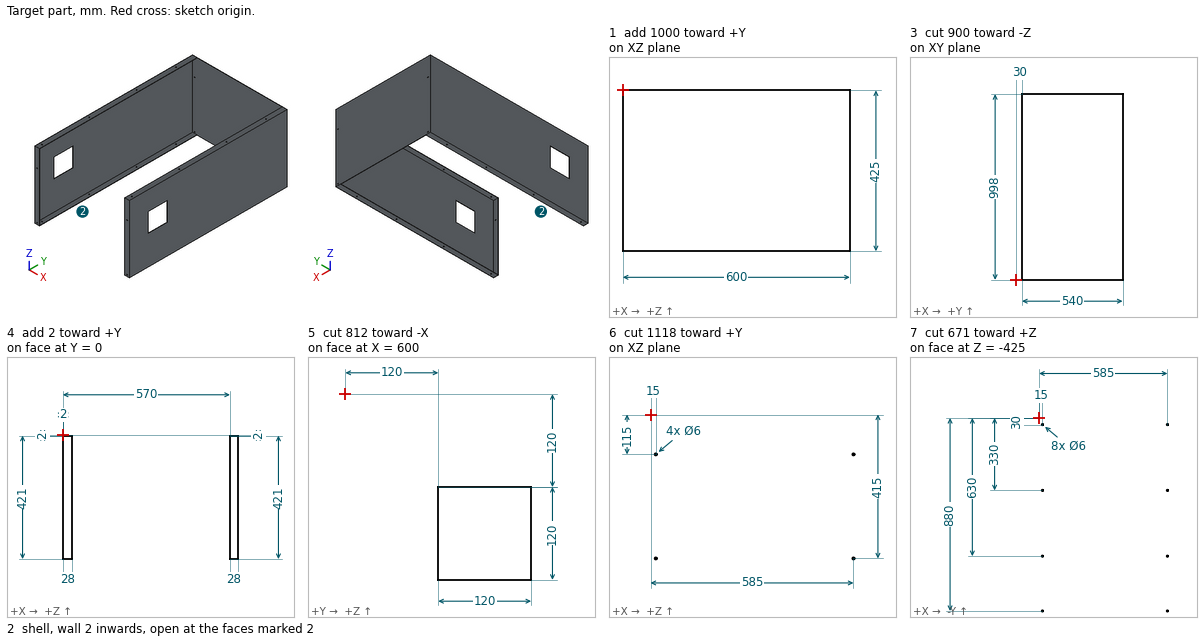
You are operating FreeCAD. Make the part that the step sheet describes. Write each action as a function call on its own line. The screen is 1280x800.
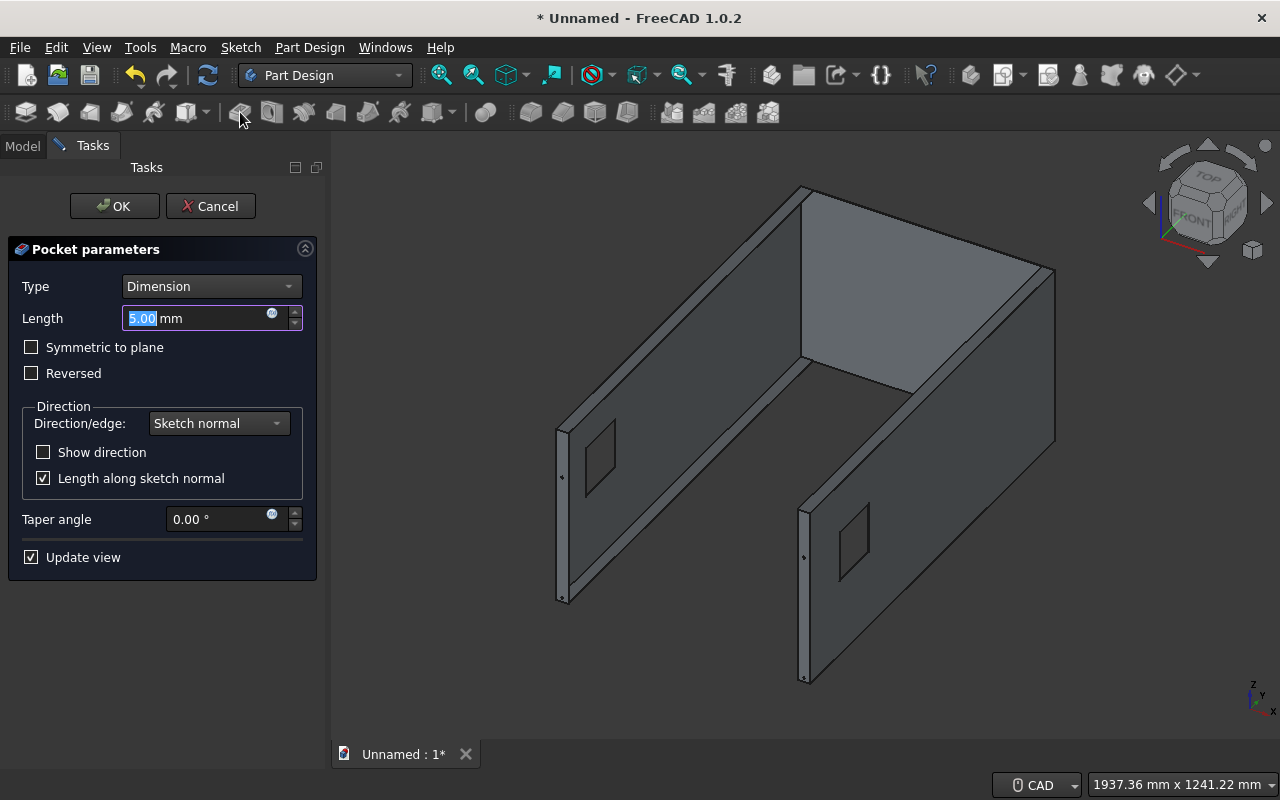
text(1118)
key(Tab)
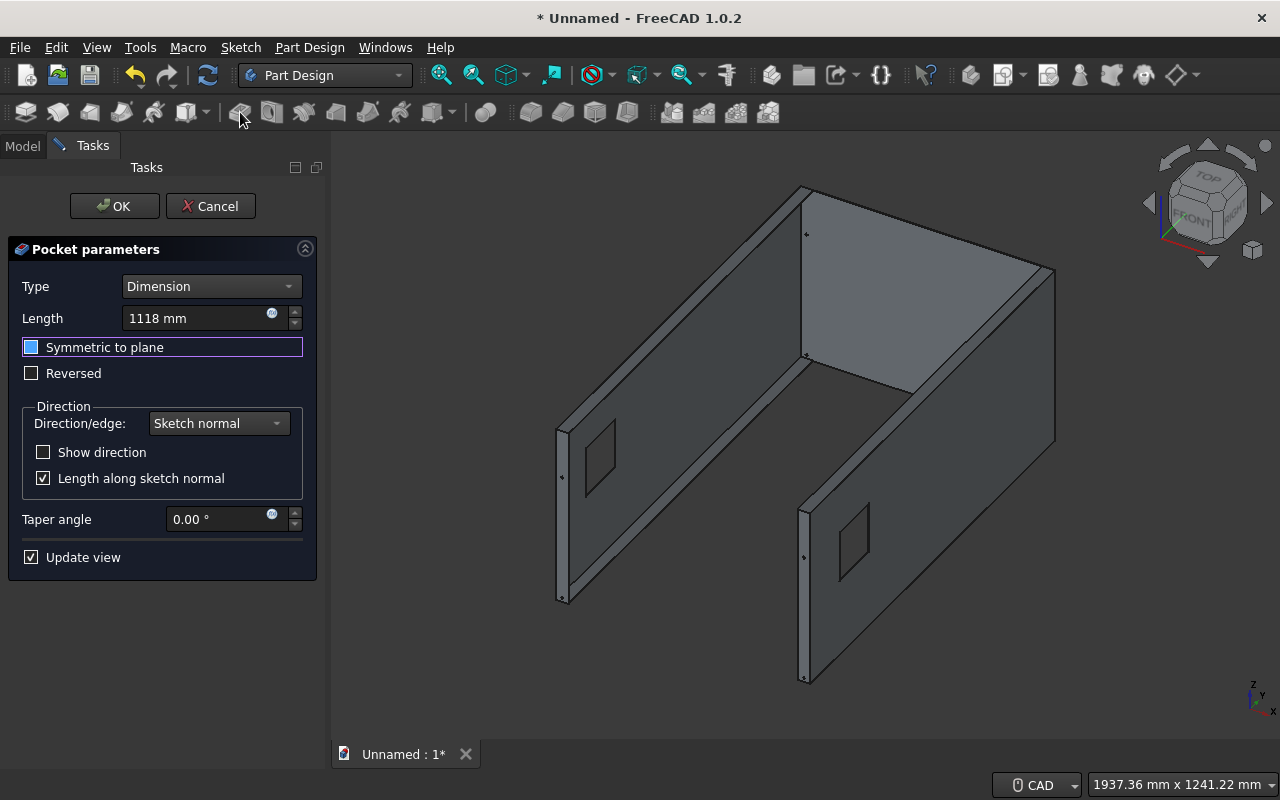
click(115, 206)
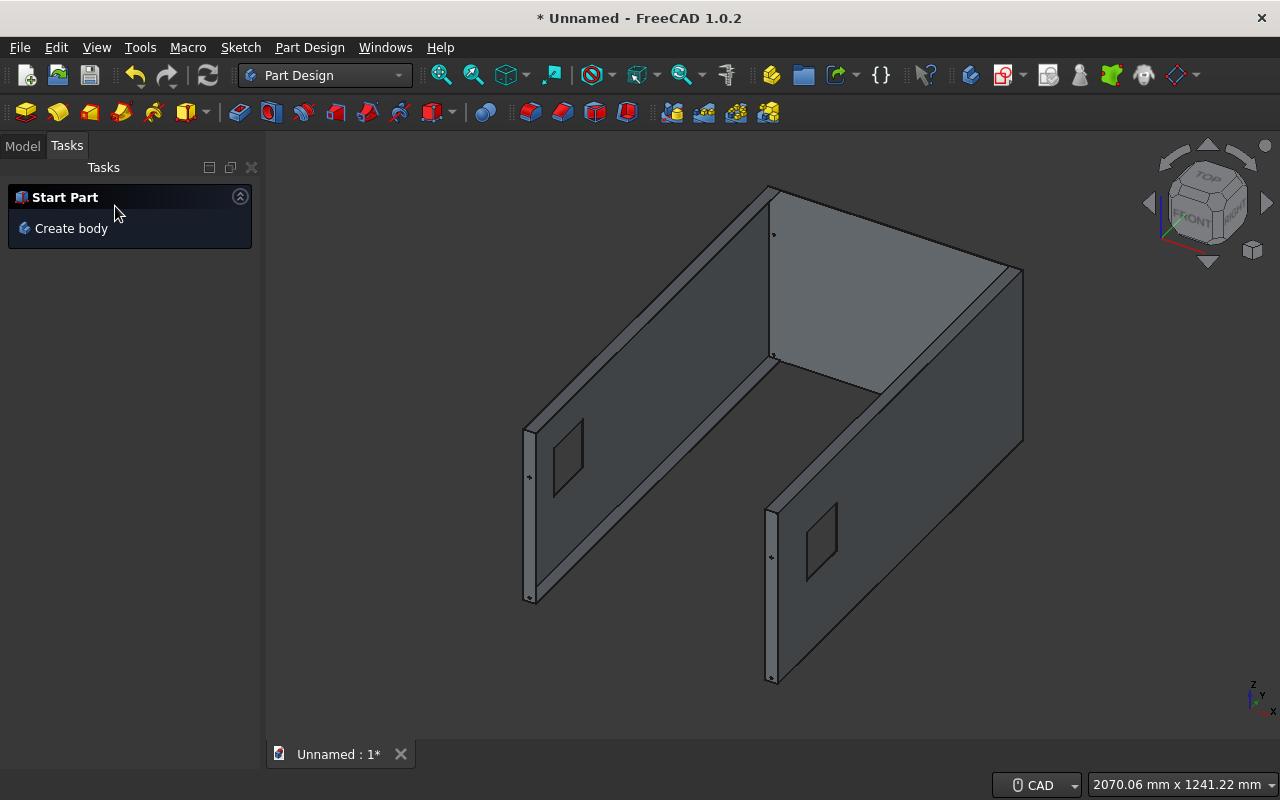
key(5)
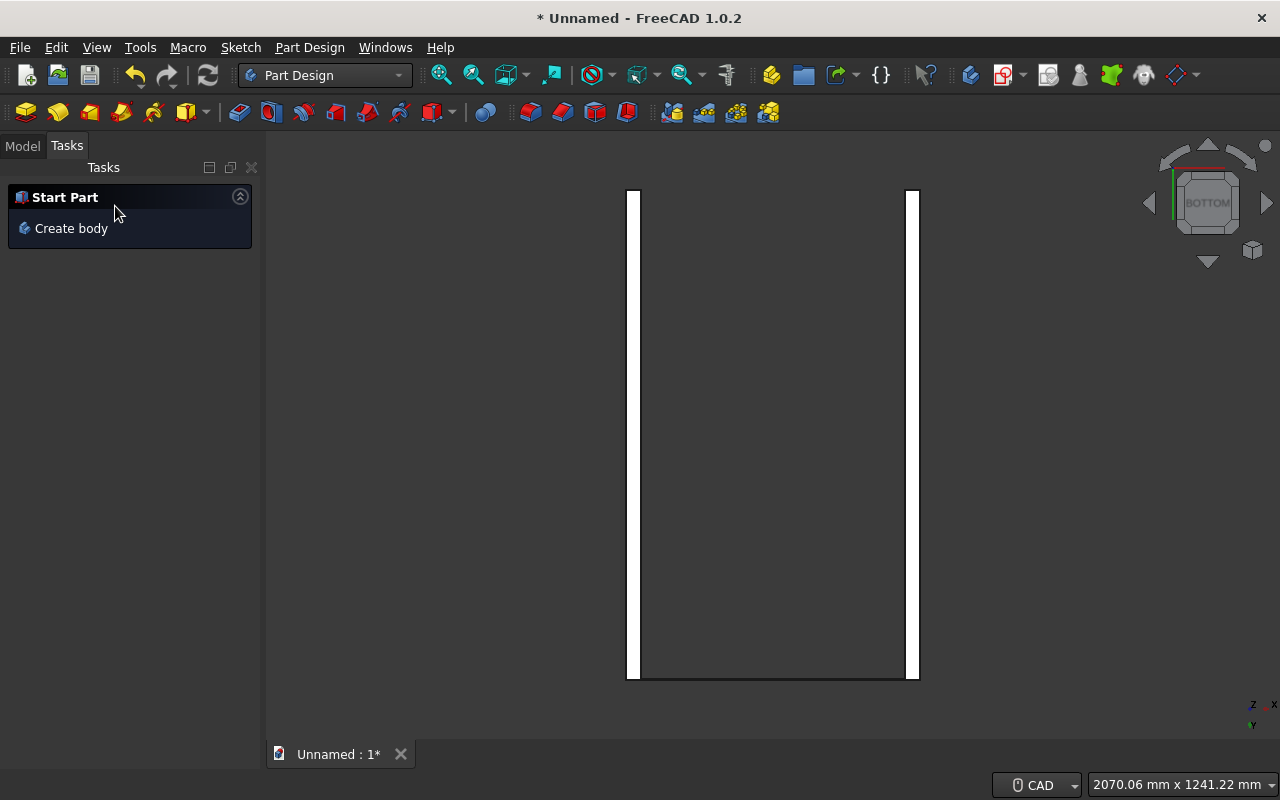
scroll(915, 515, up, 5)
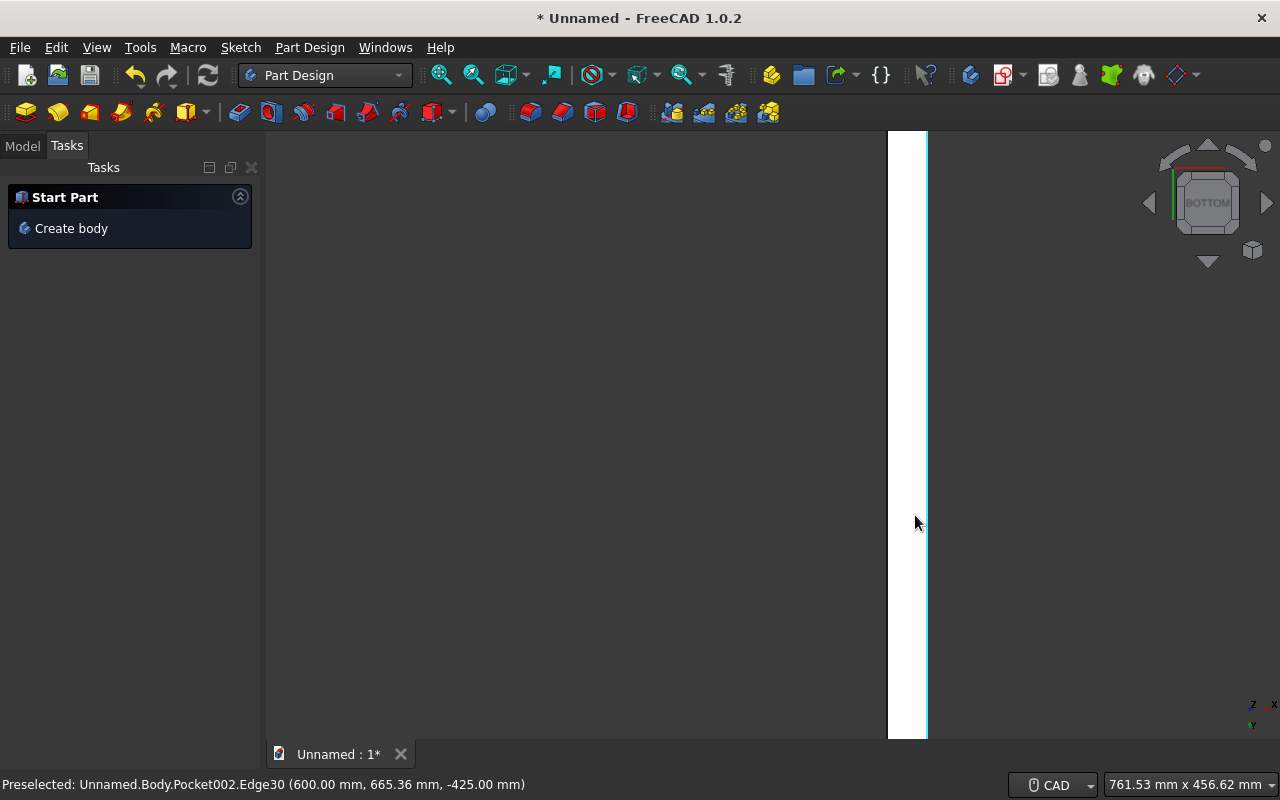
click(914, 516)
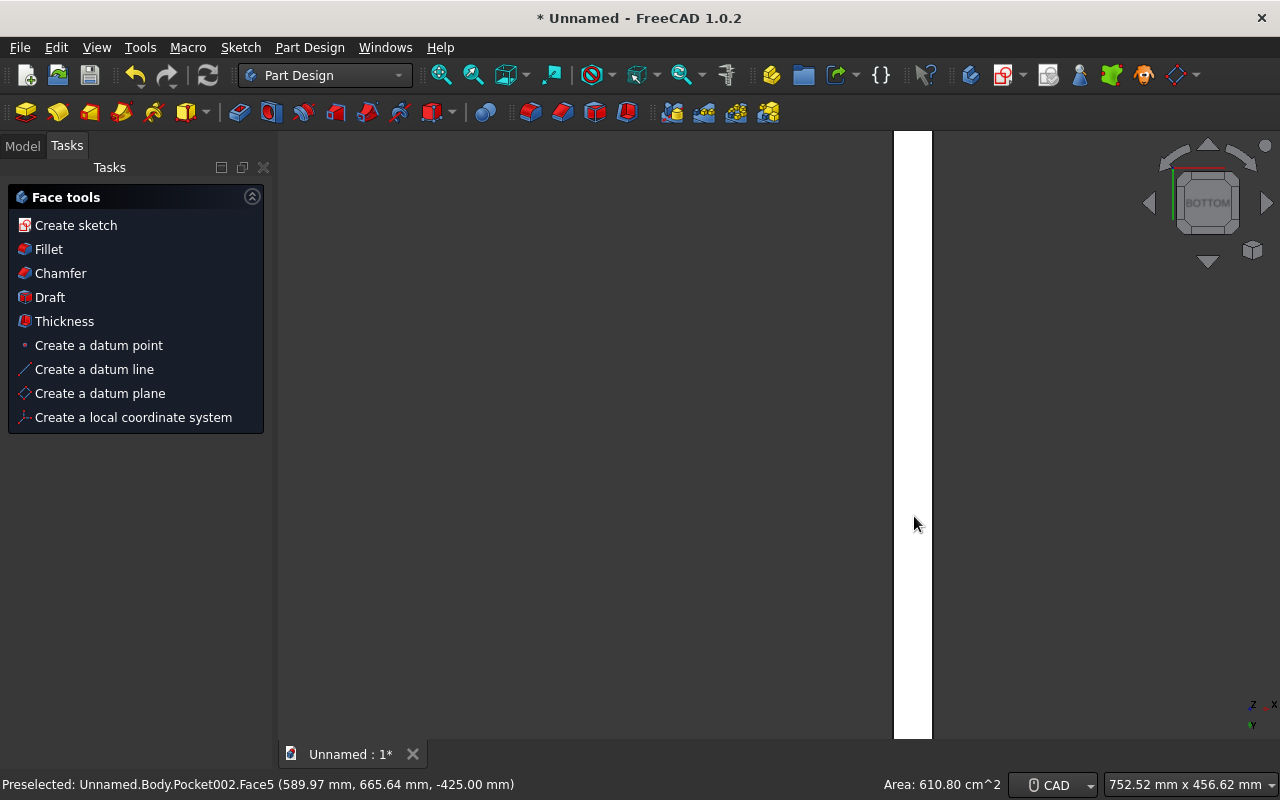
click(1004, 76)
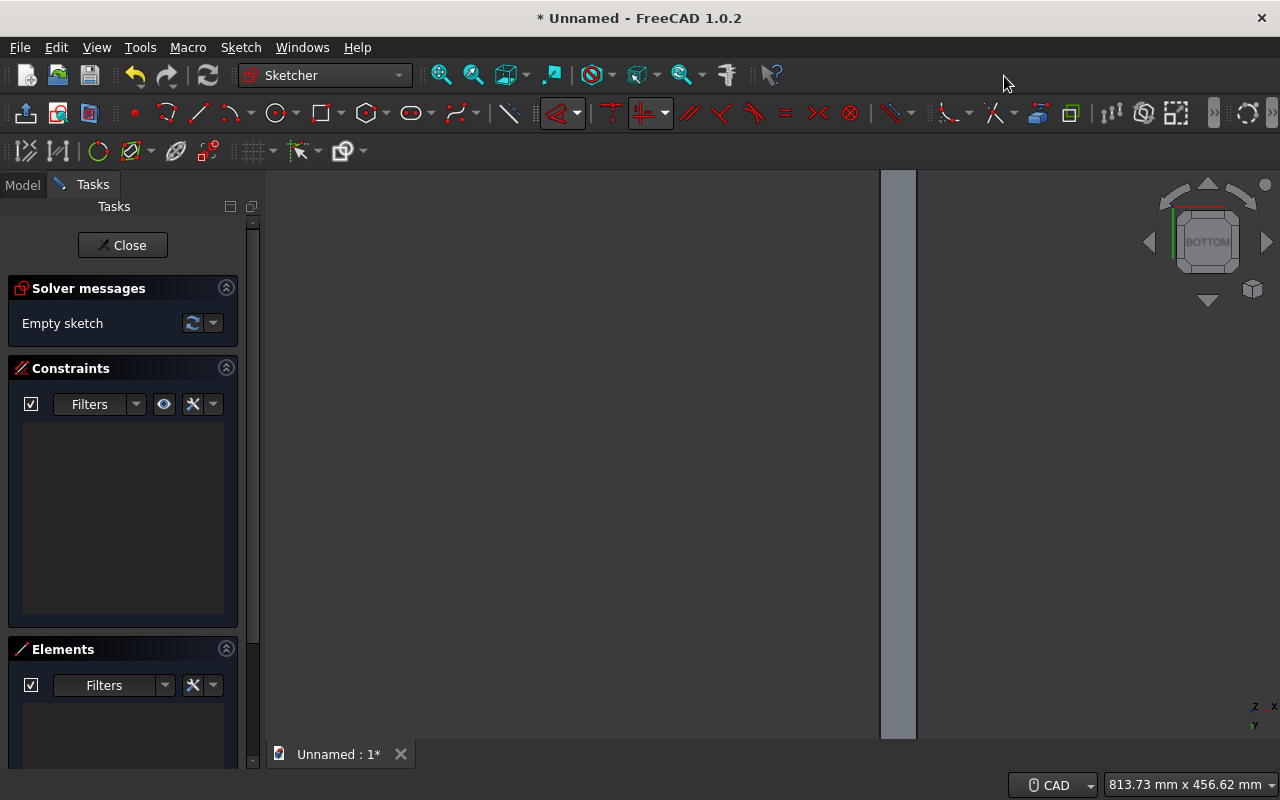
scroll(777, 542, down, 6)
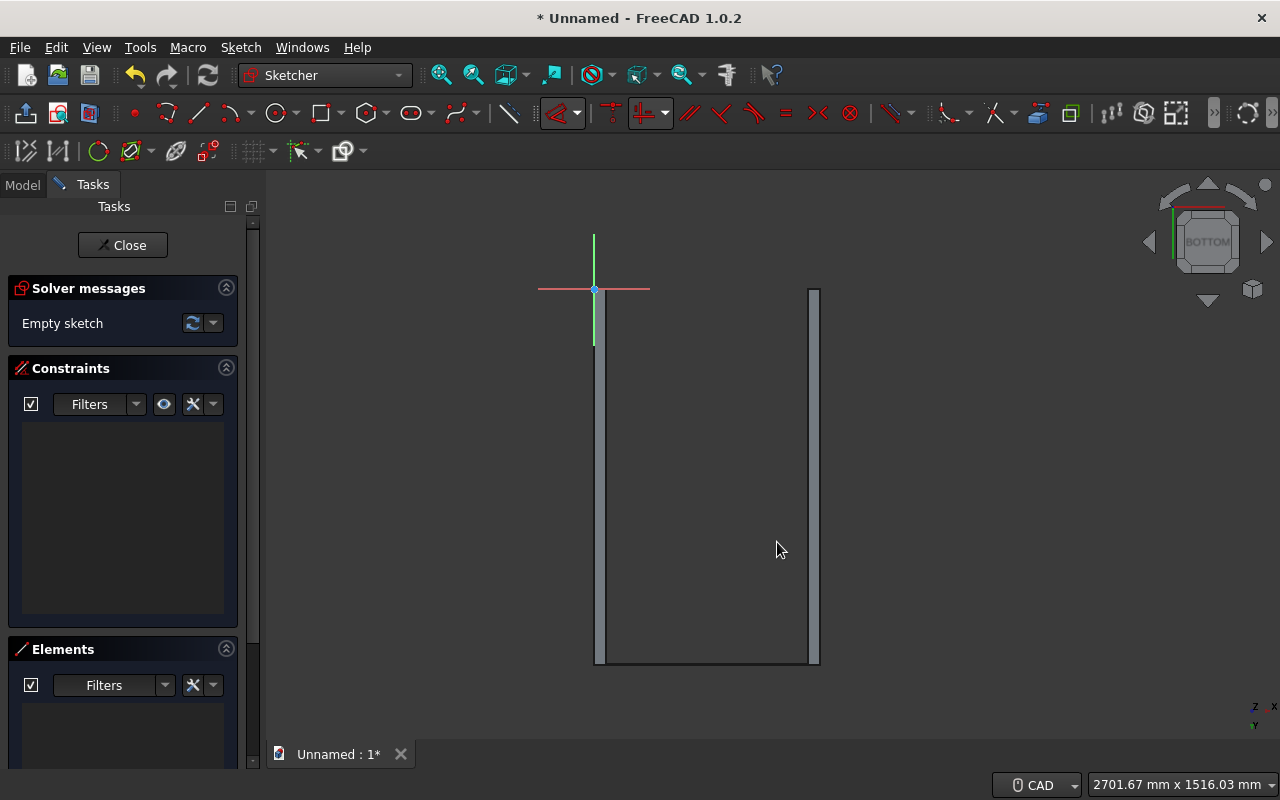
click(276, 114)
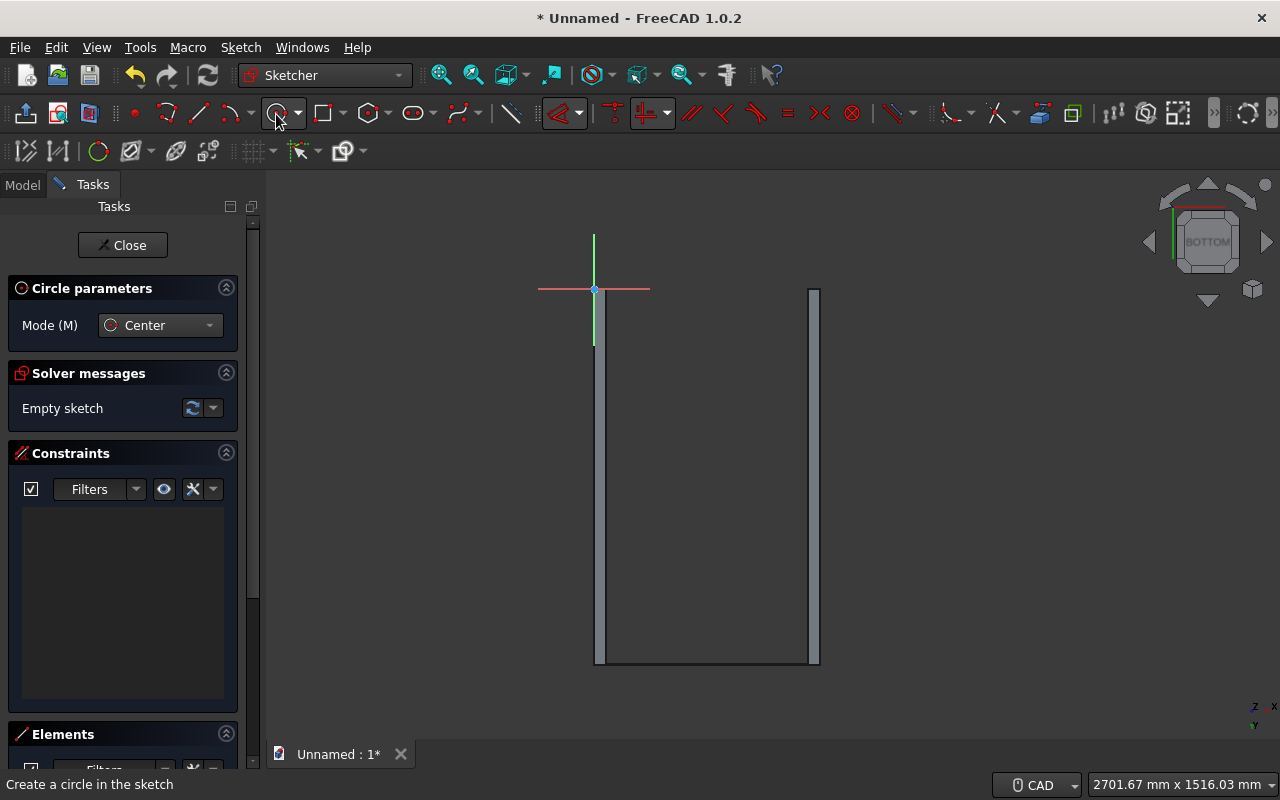
scroll(600, 301, up, 16)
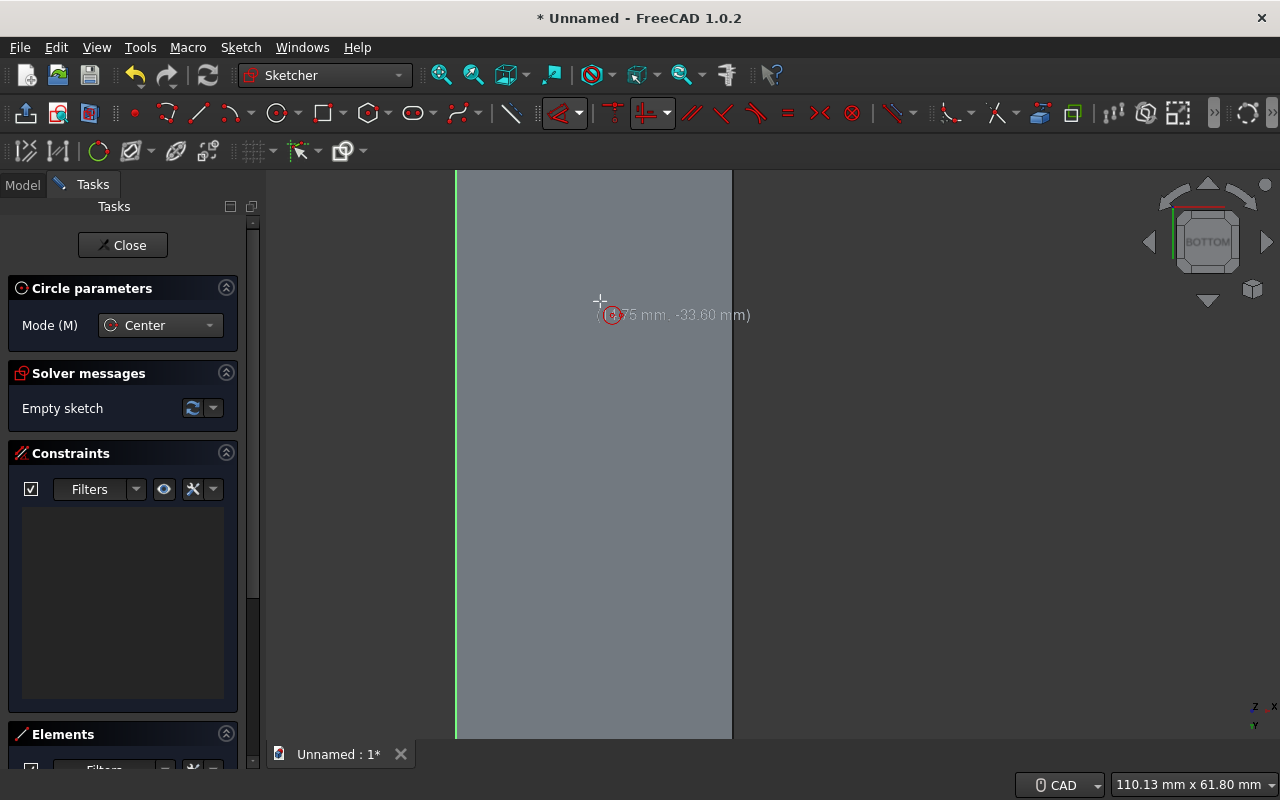
scroll(576, 265, down, 15)